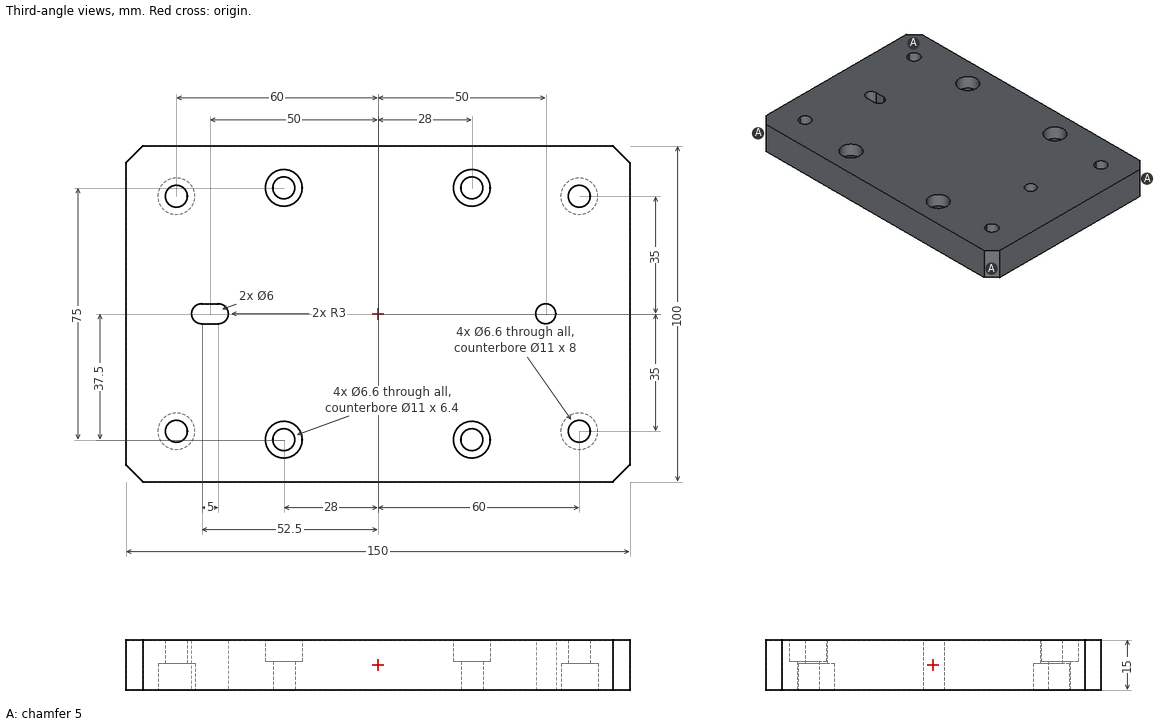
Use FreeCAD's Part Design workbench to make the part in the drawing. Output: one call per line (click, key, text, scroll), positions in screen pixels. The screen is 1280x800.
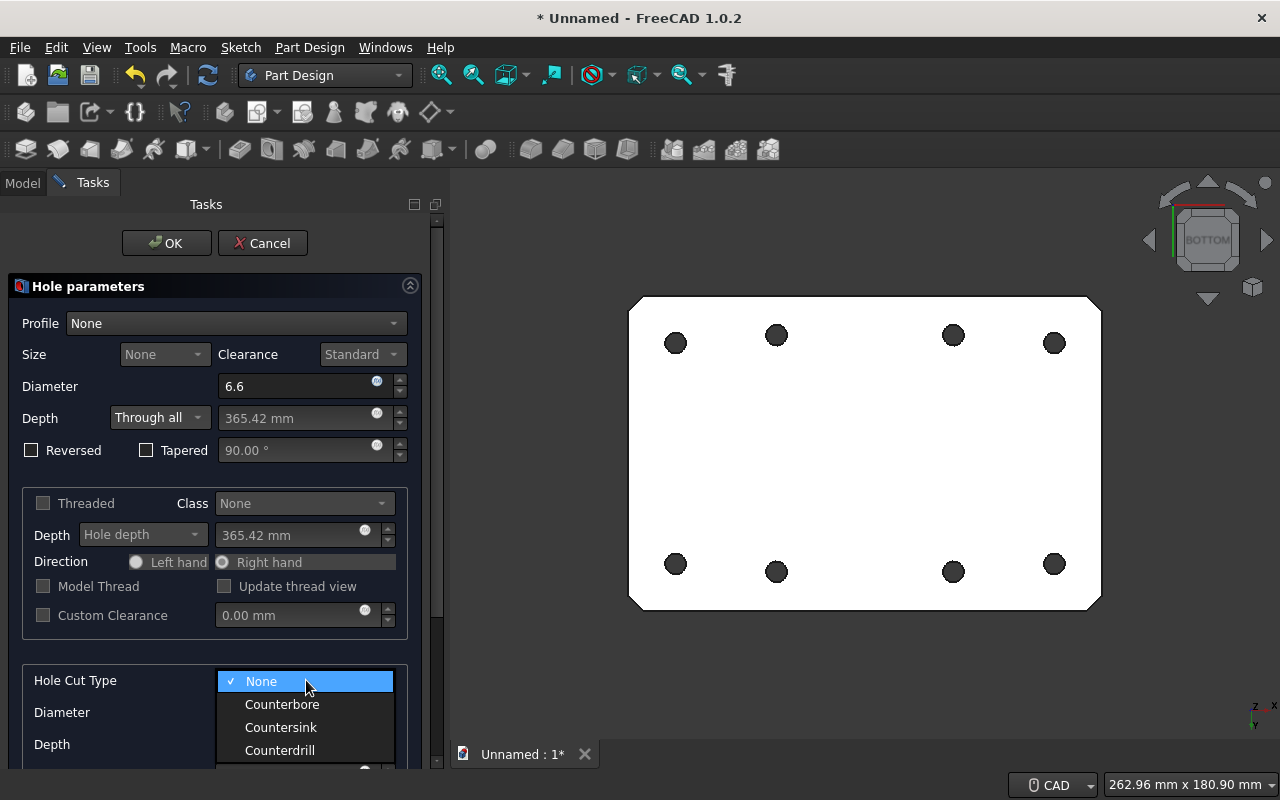
click(304, 704)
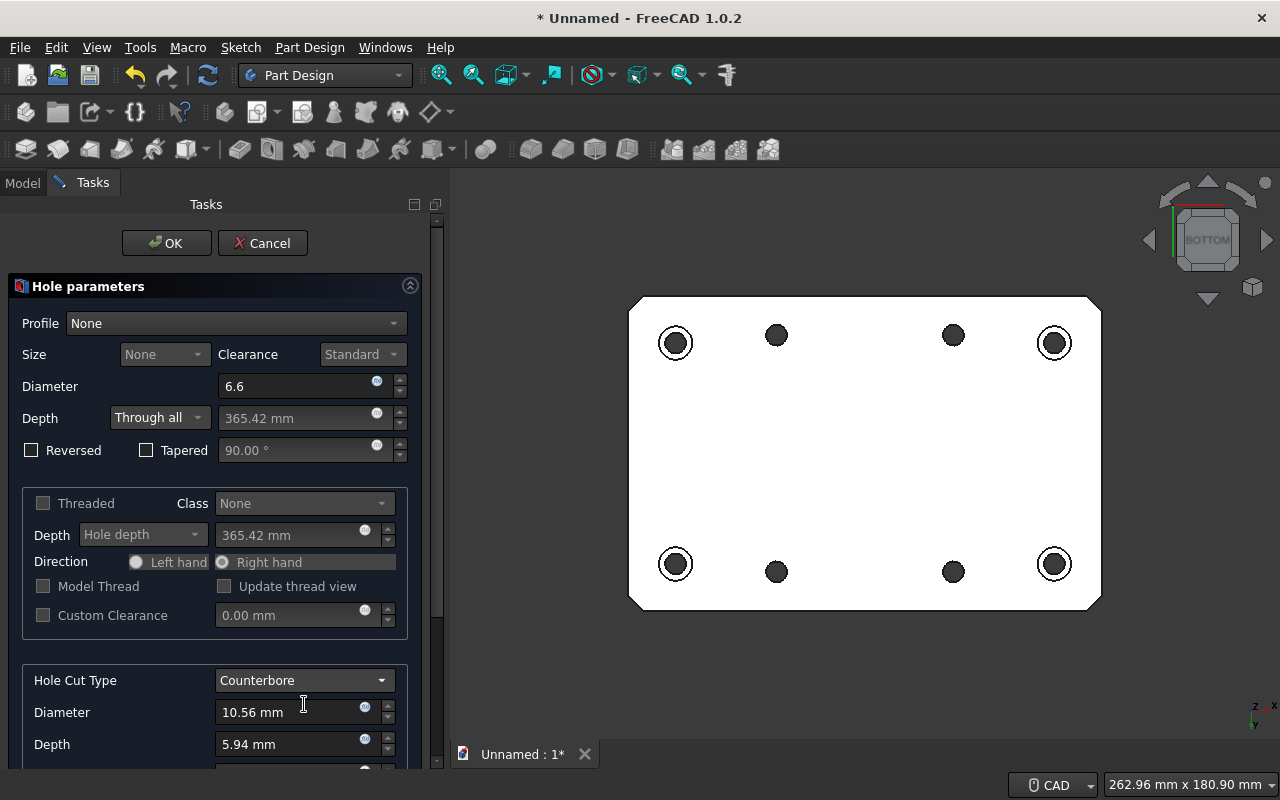
triple_click(298, 712)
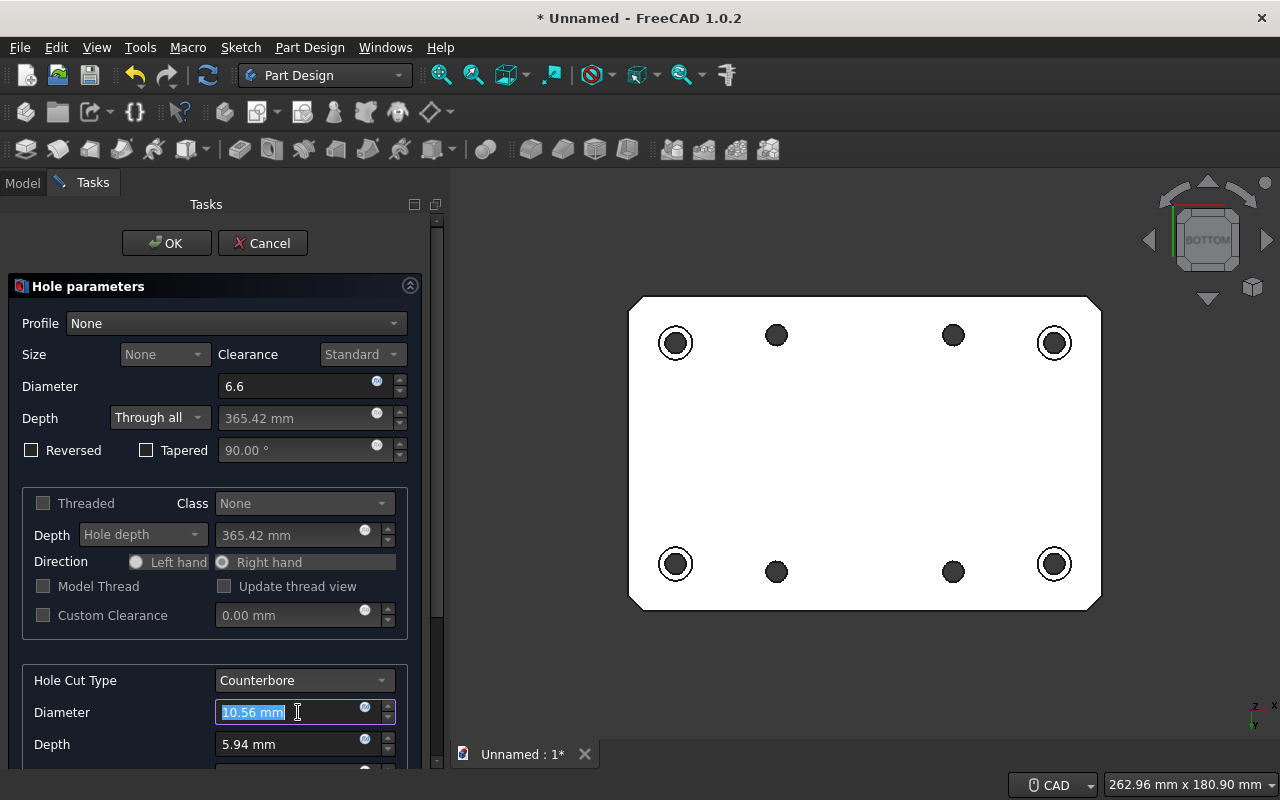
text(11)
key(Tab)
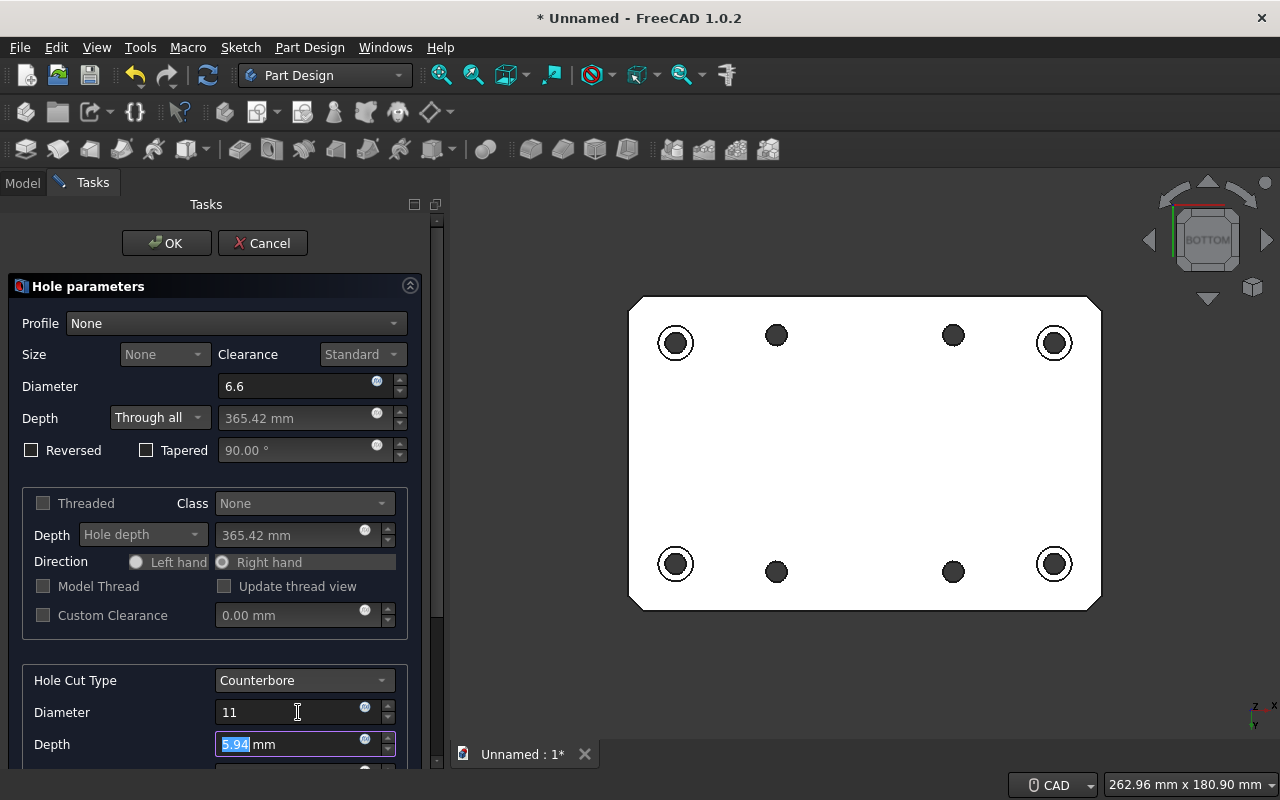
text(8)
key(Tab)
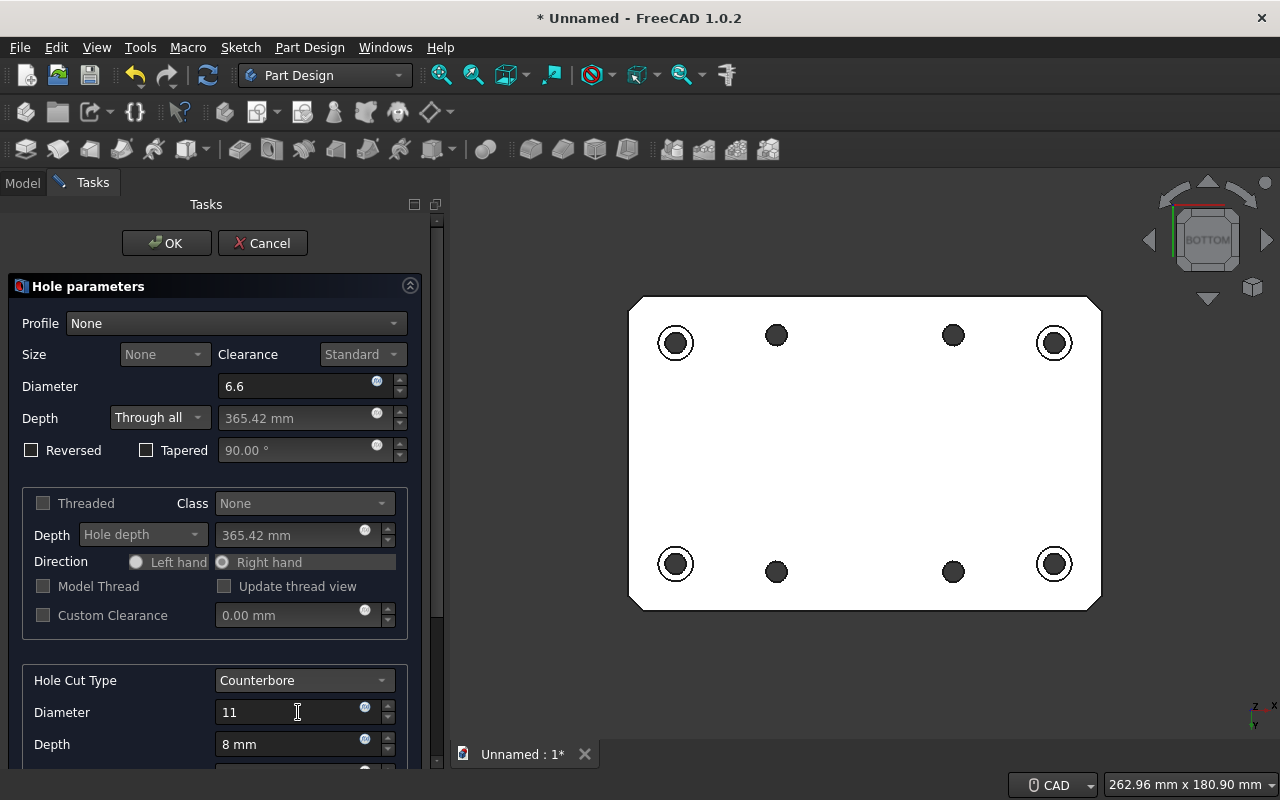
click(167, 243)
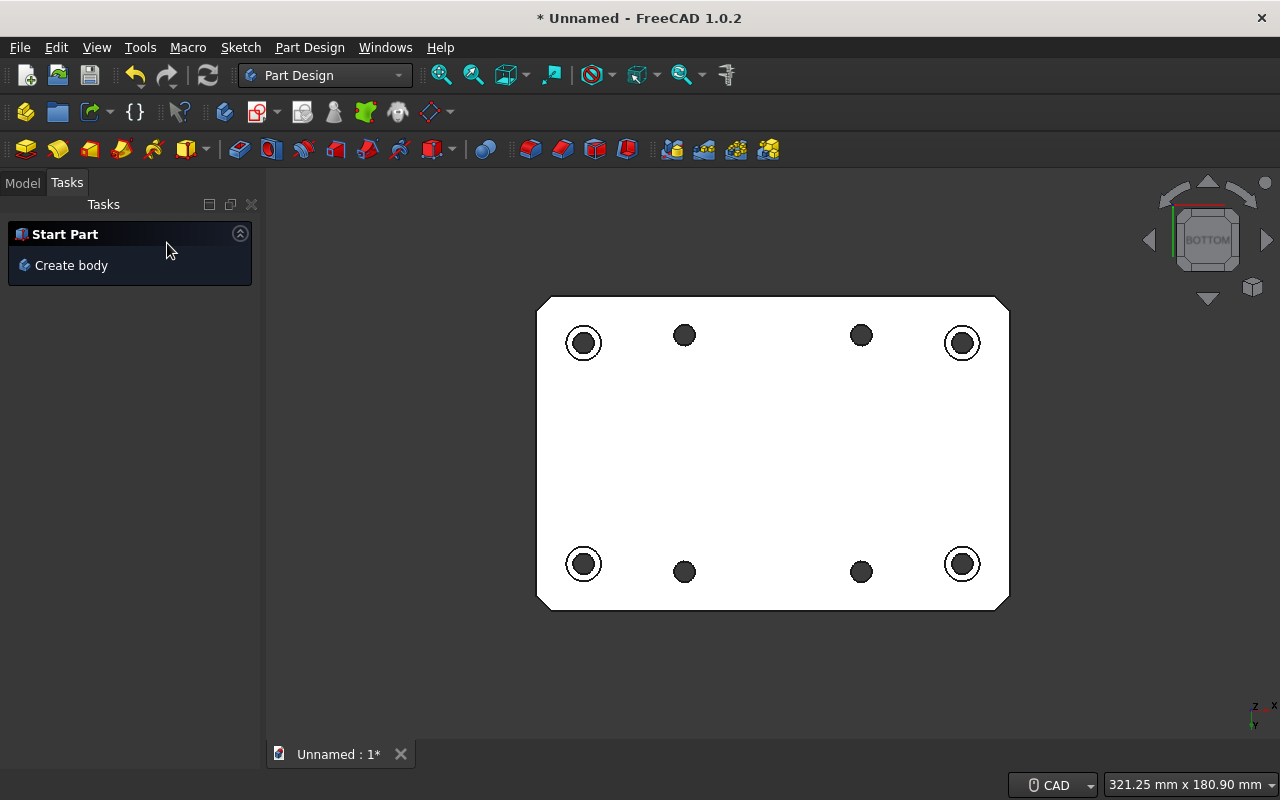
click(773, 453)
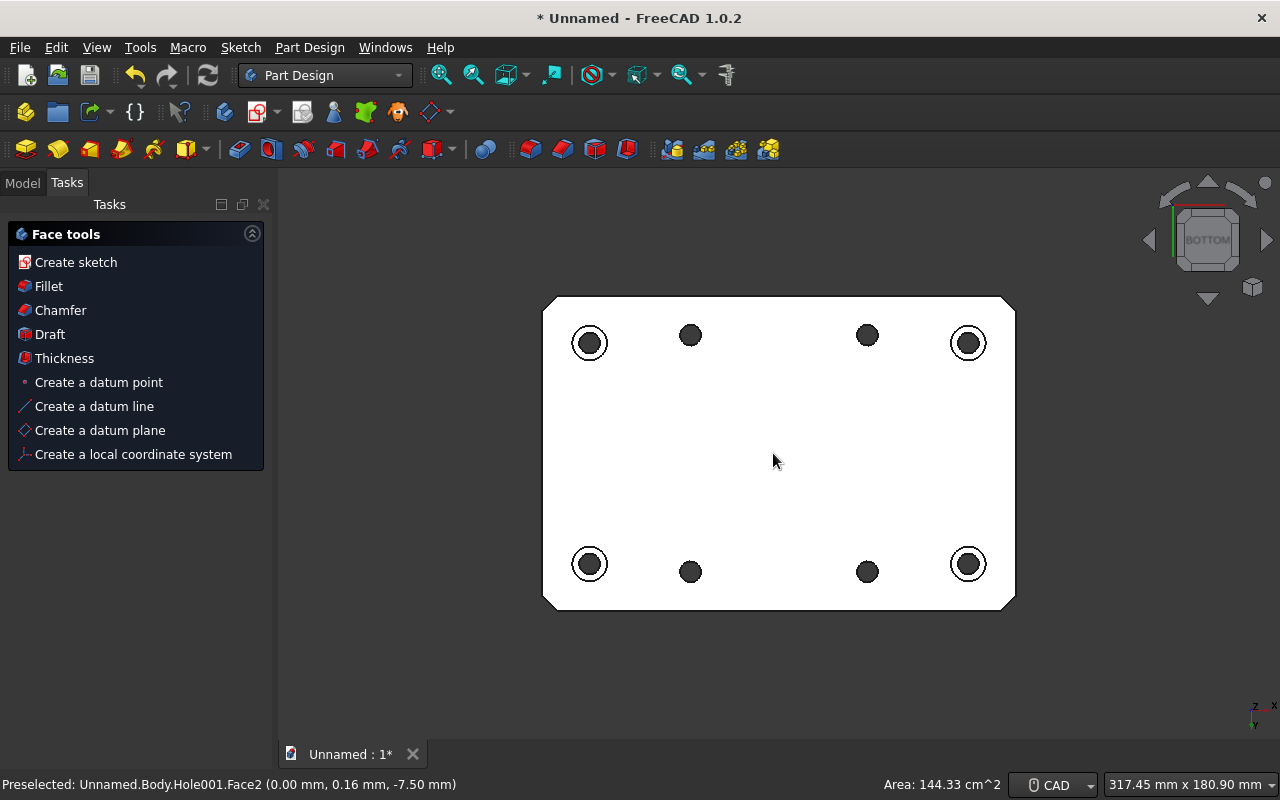
click(258, 112)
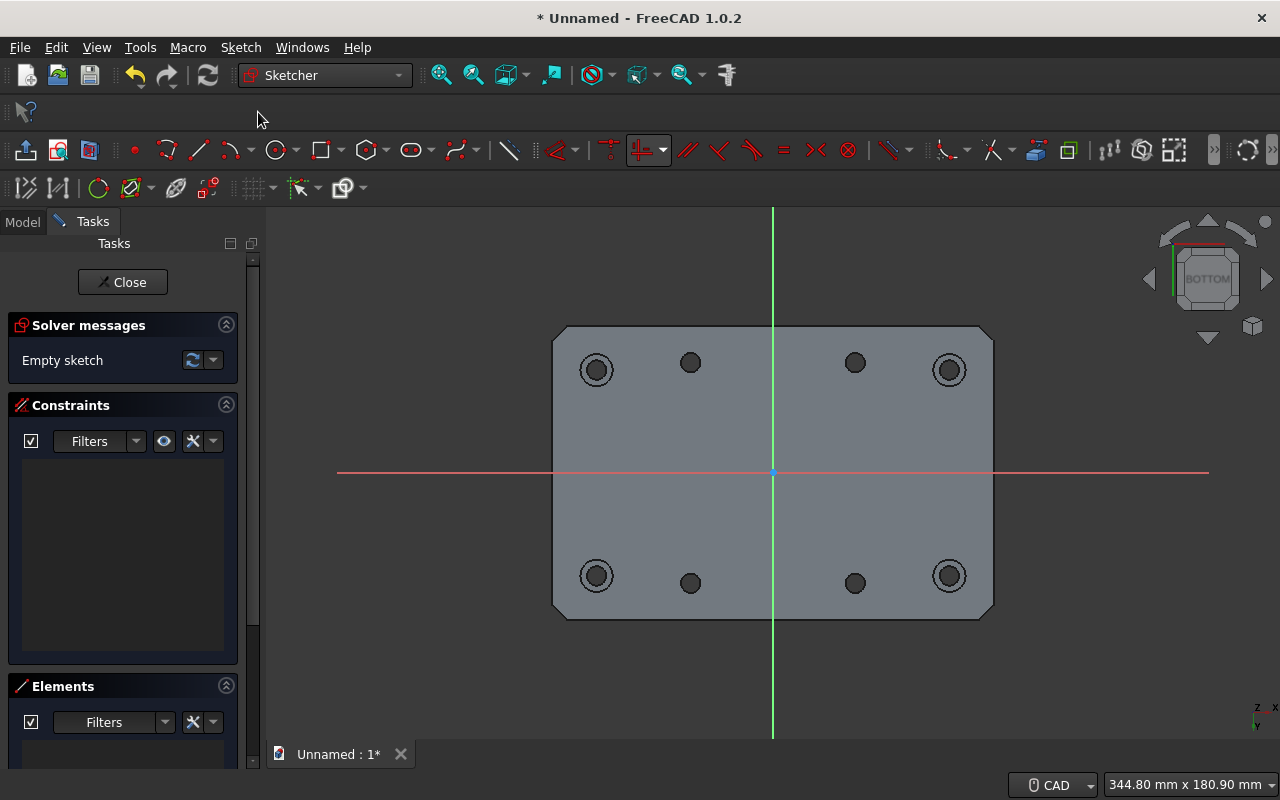
scroll(856, 473, up, 3)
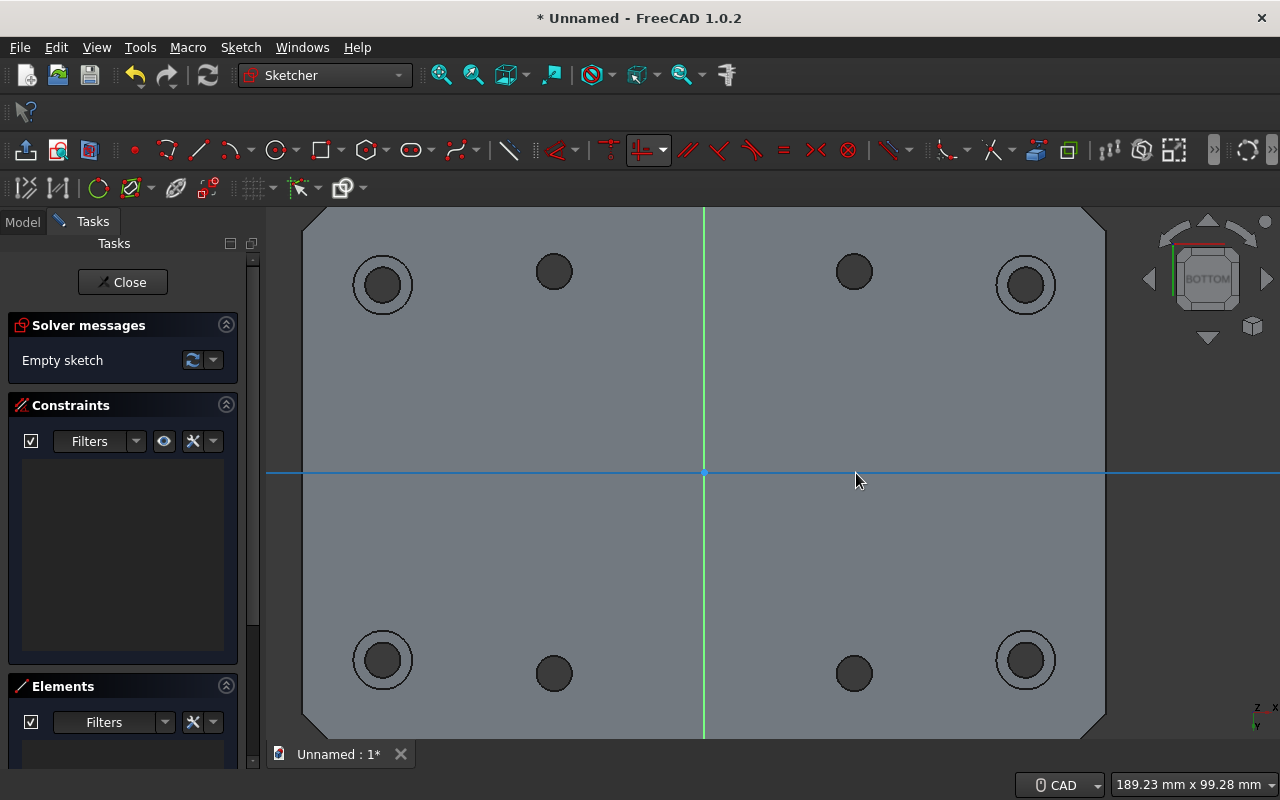
key(g)
key(c)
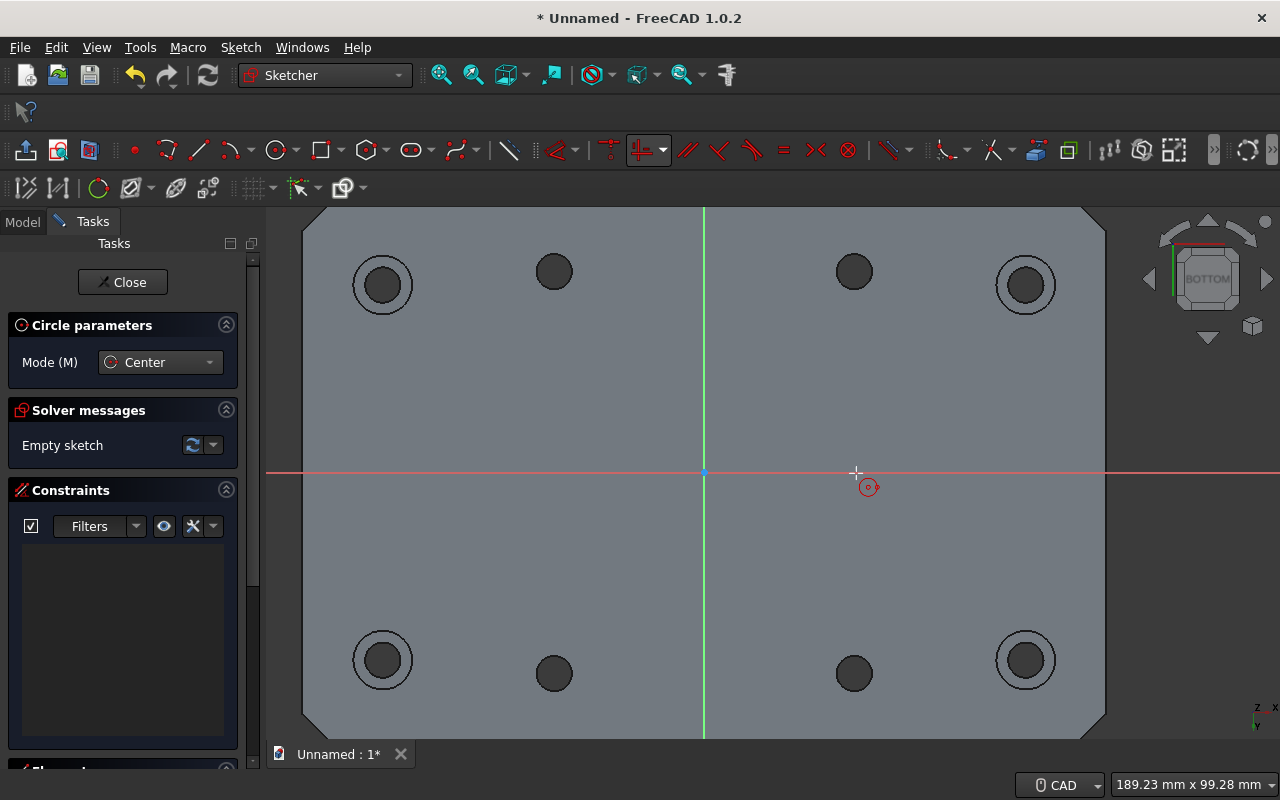
scroll(436, 473, up, 2)